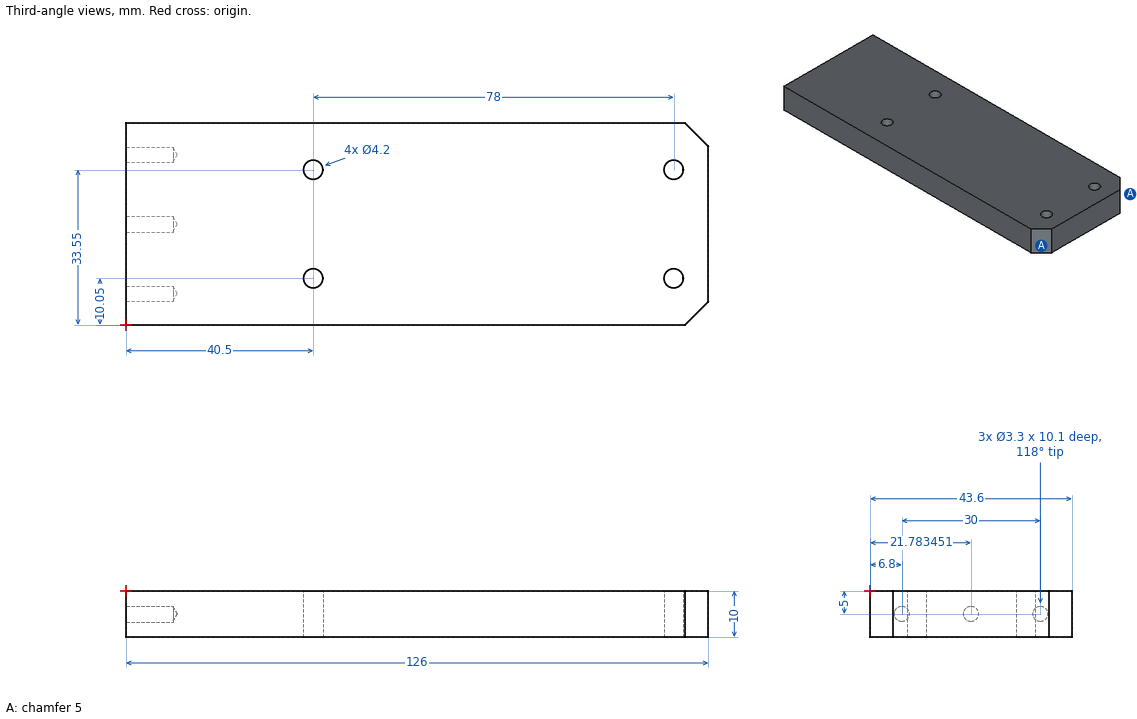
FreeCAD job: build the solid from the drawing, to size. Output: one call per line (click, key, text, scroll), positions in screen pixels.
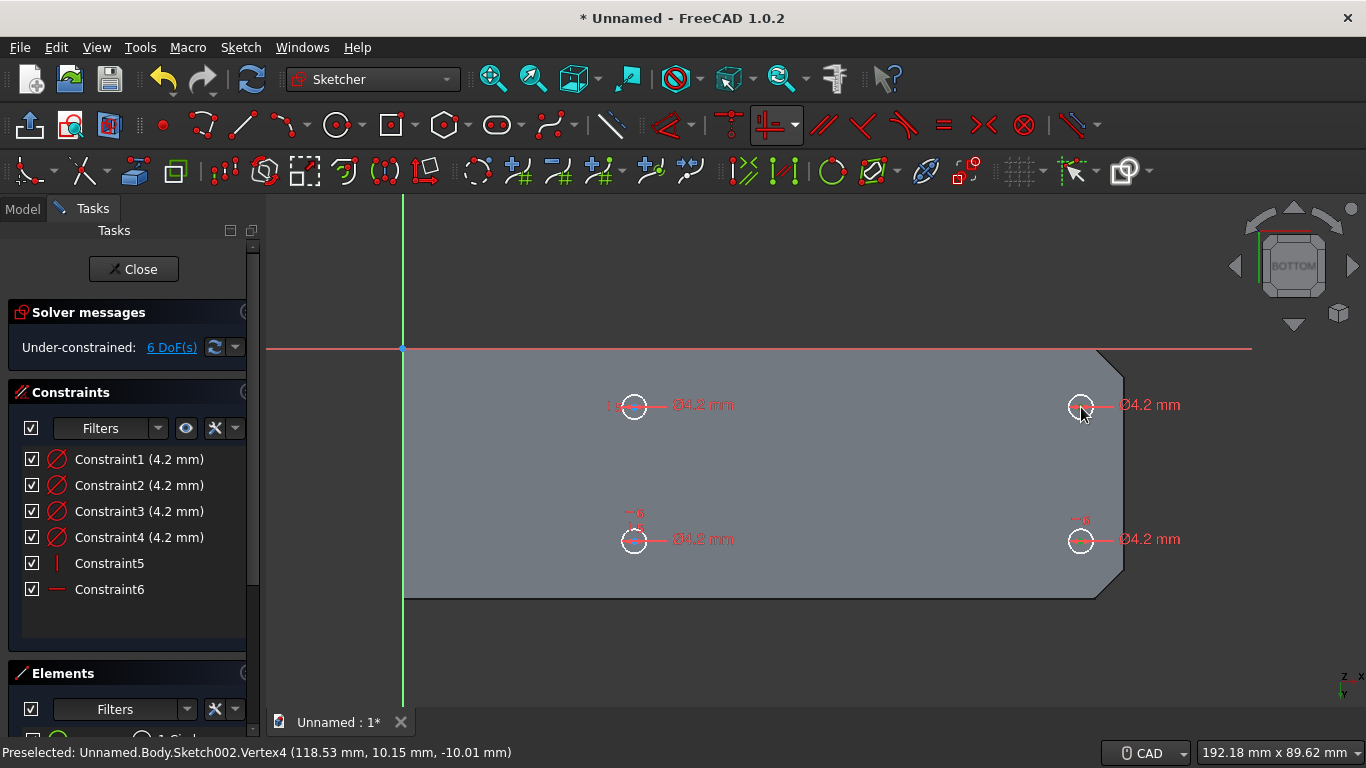
key(v)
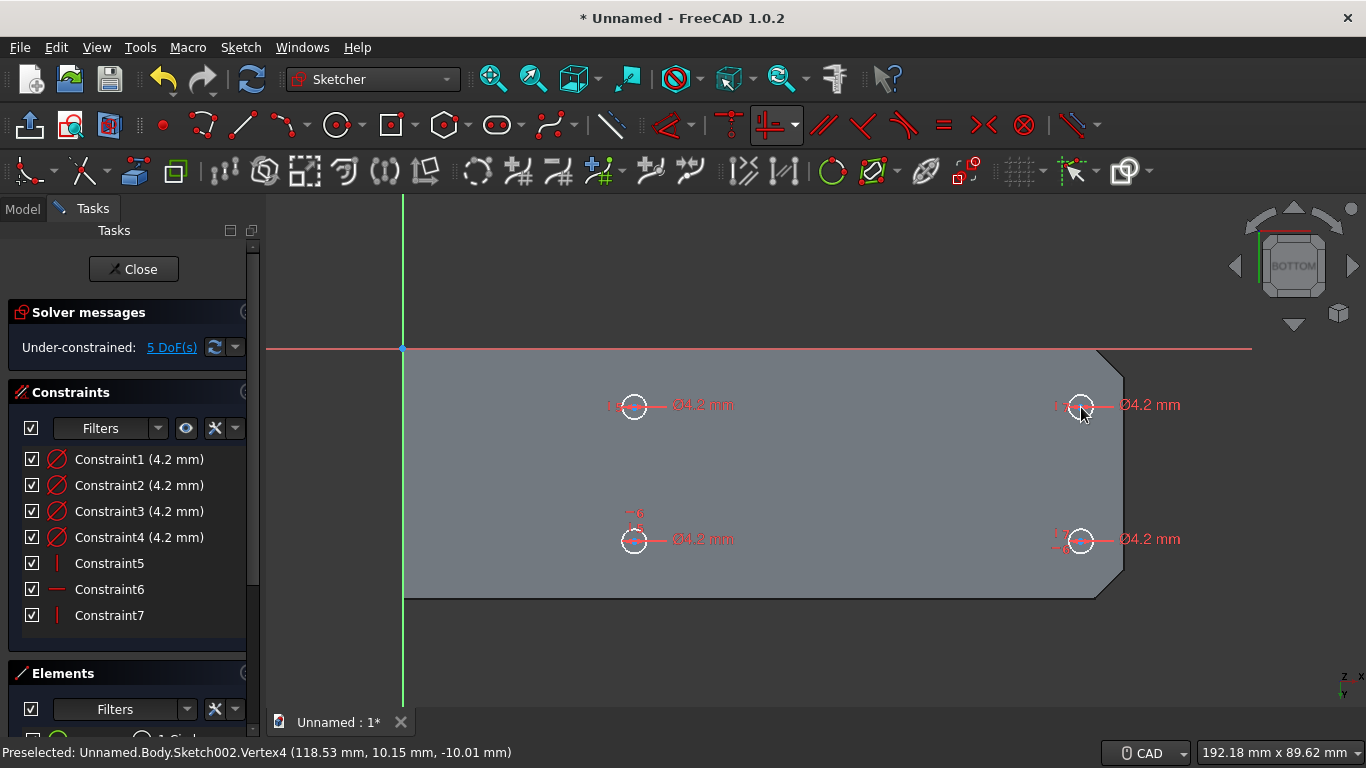
click(634, 407)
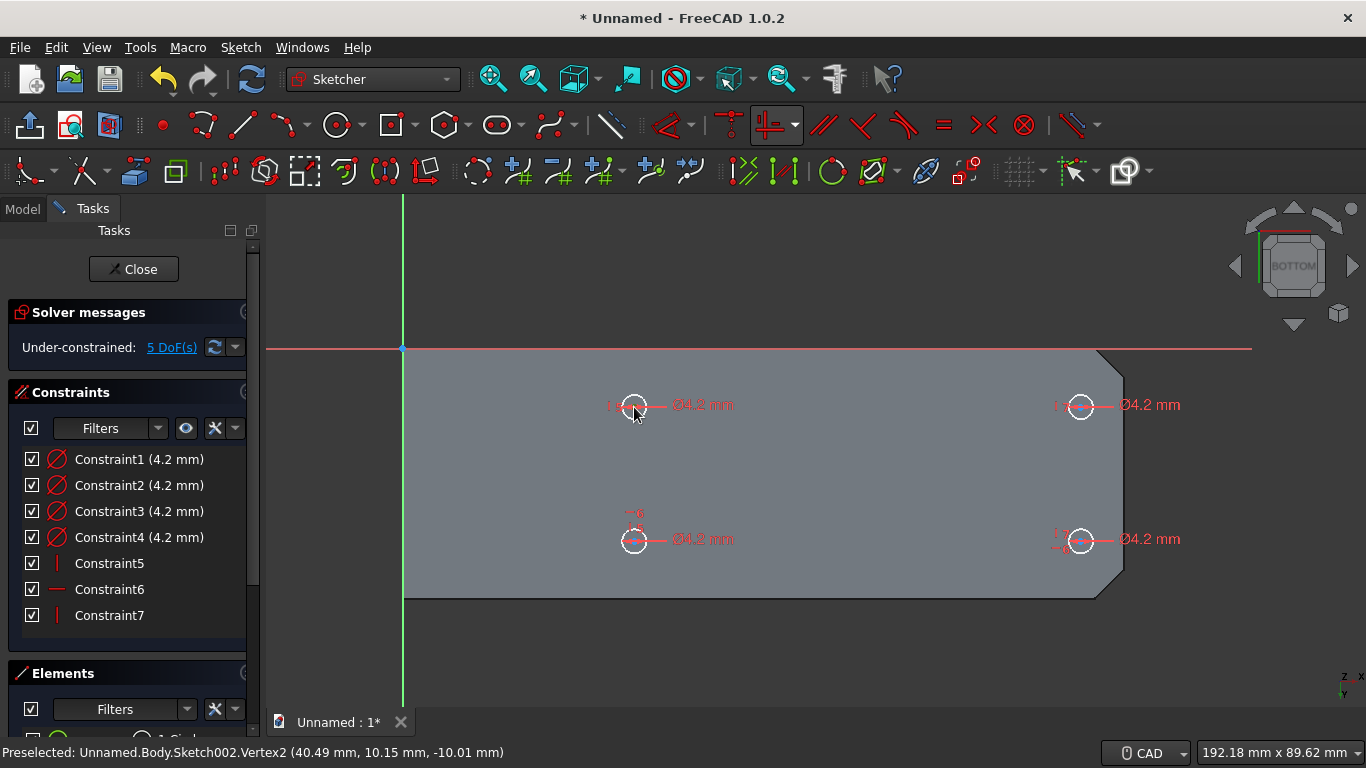
click(1081, 407)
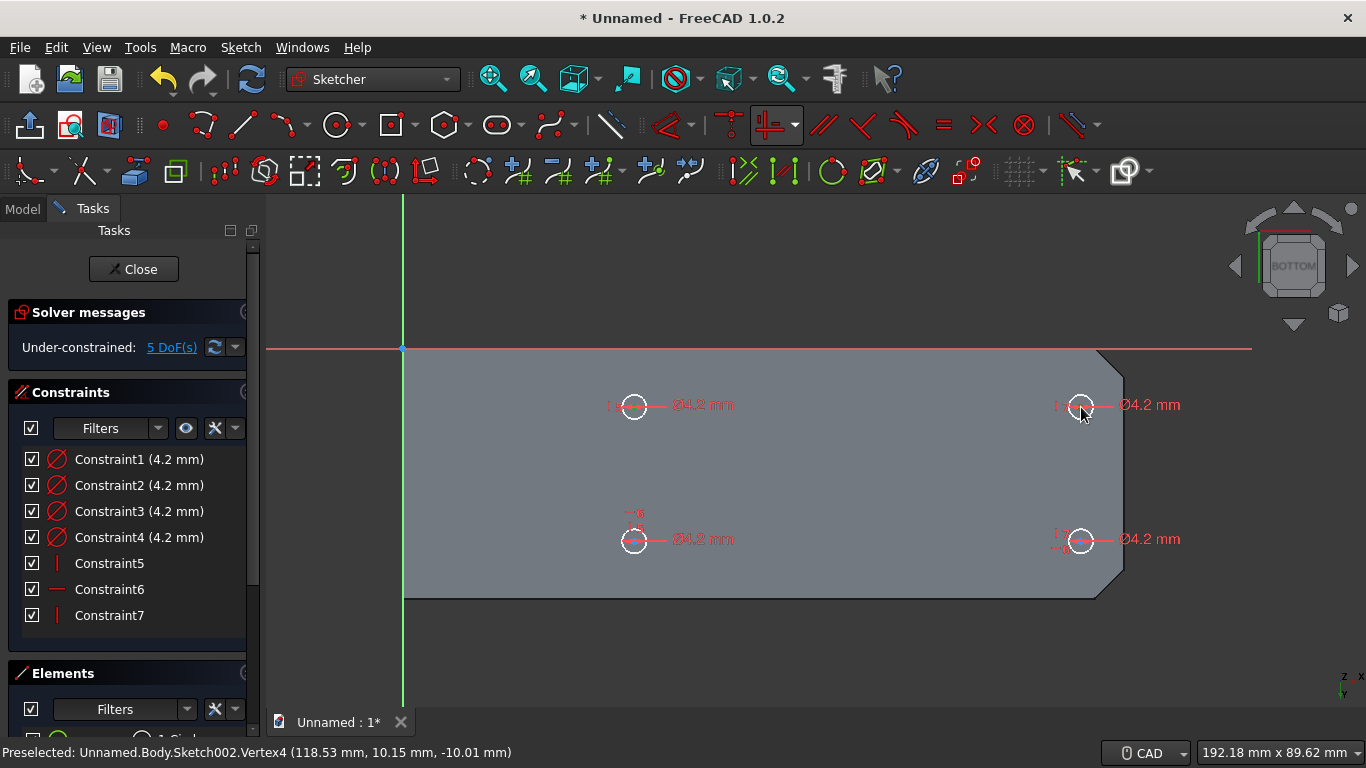
click(798, 126)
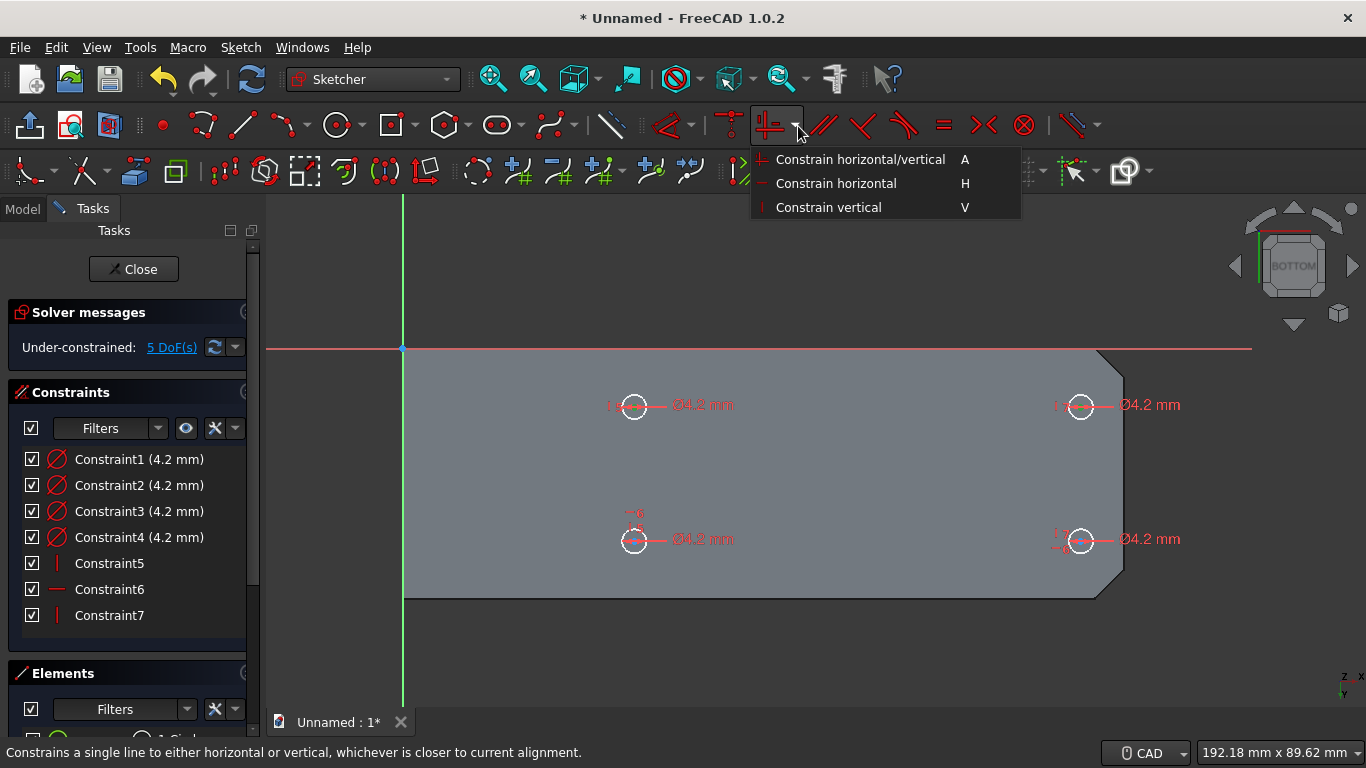
click(886, 183)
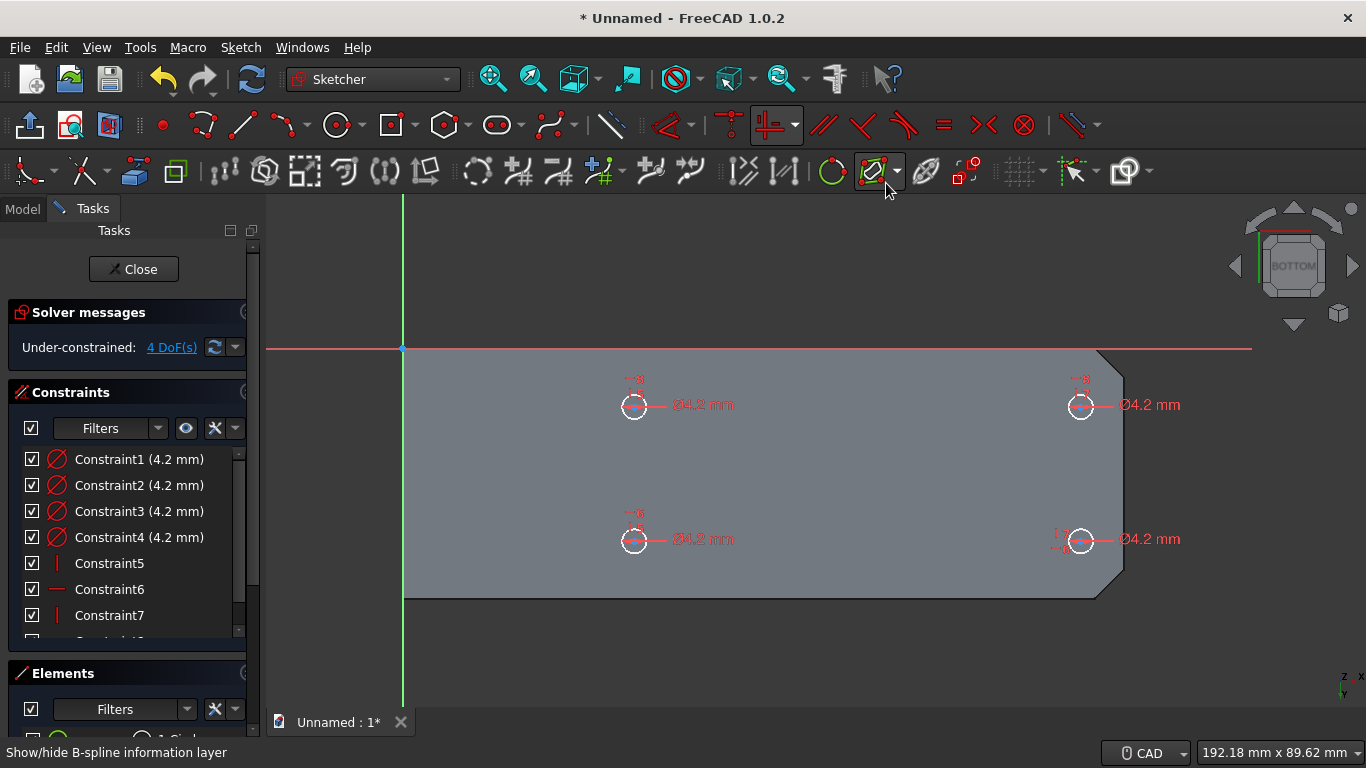
click(666, 126)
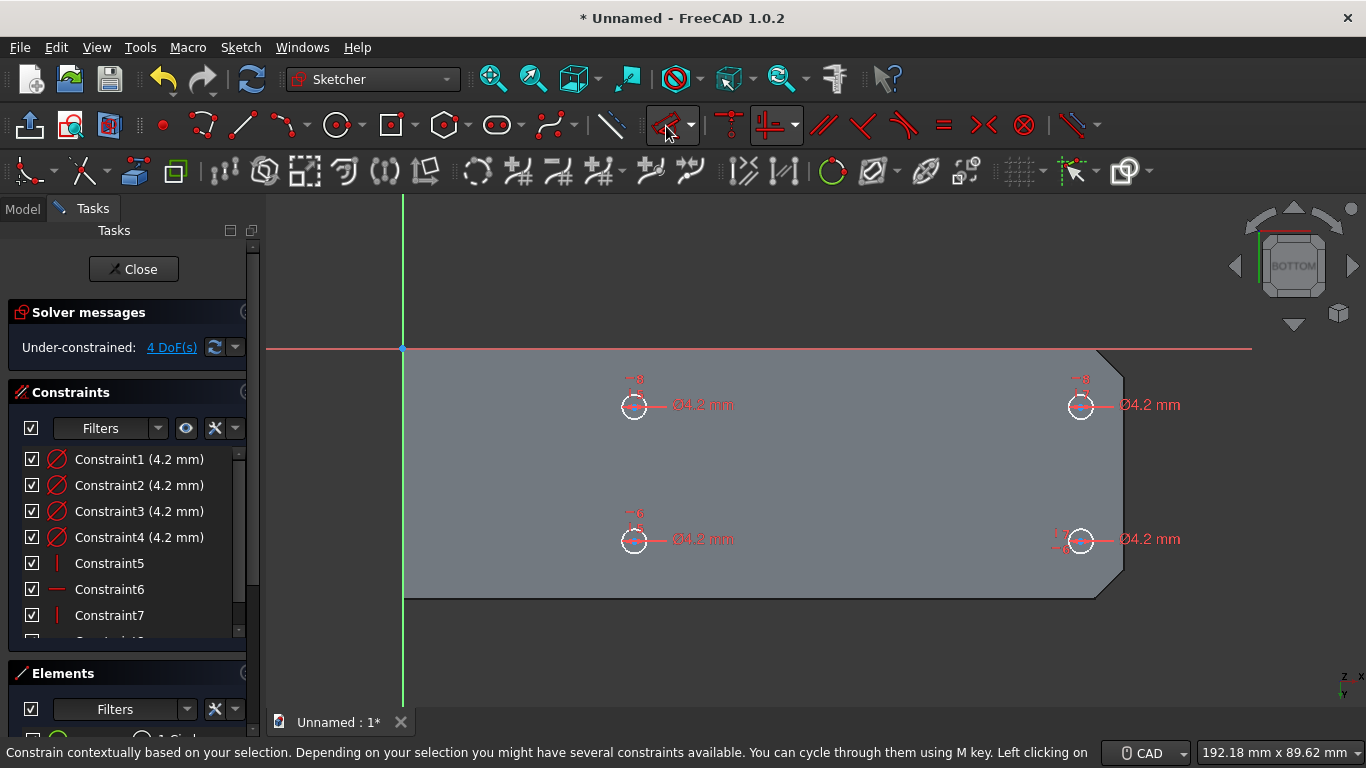
click(634, 541)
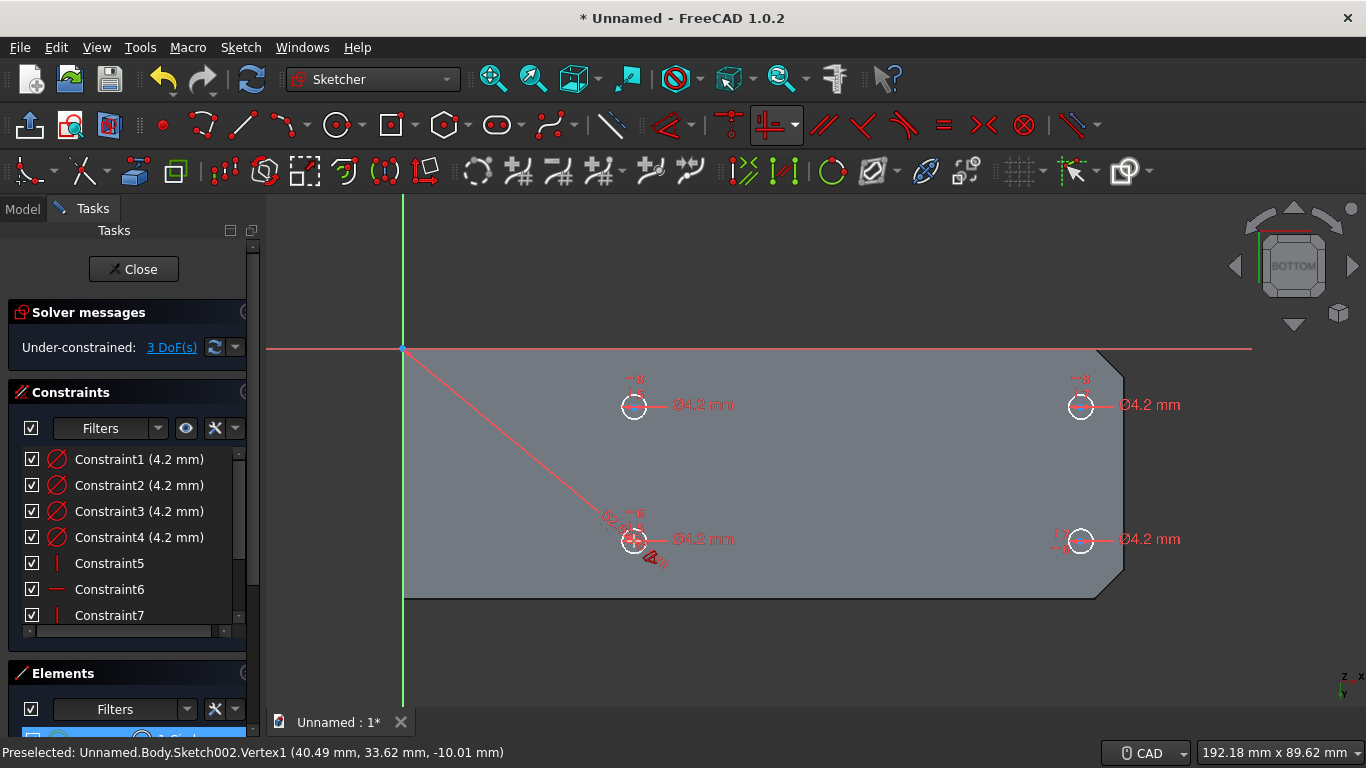
click(1081, 541)
click(858, 575)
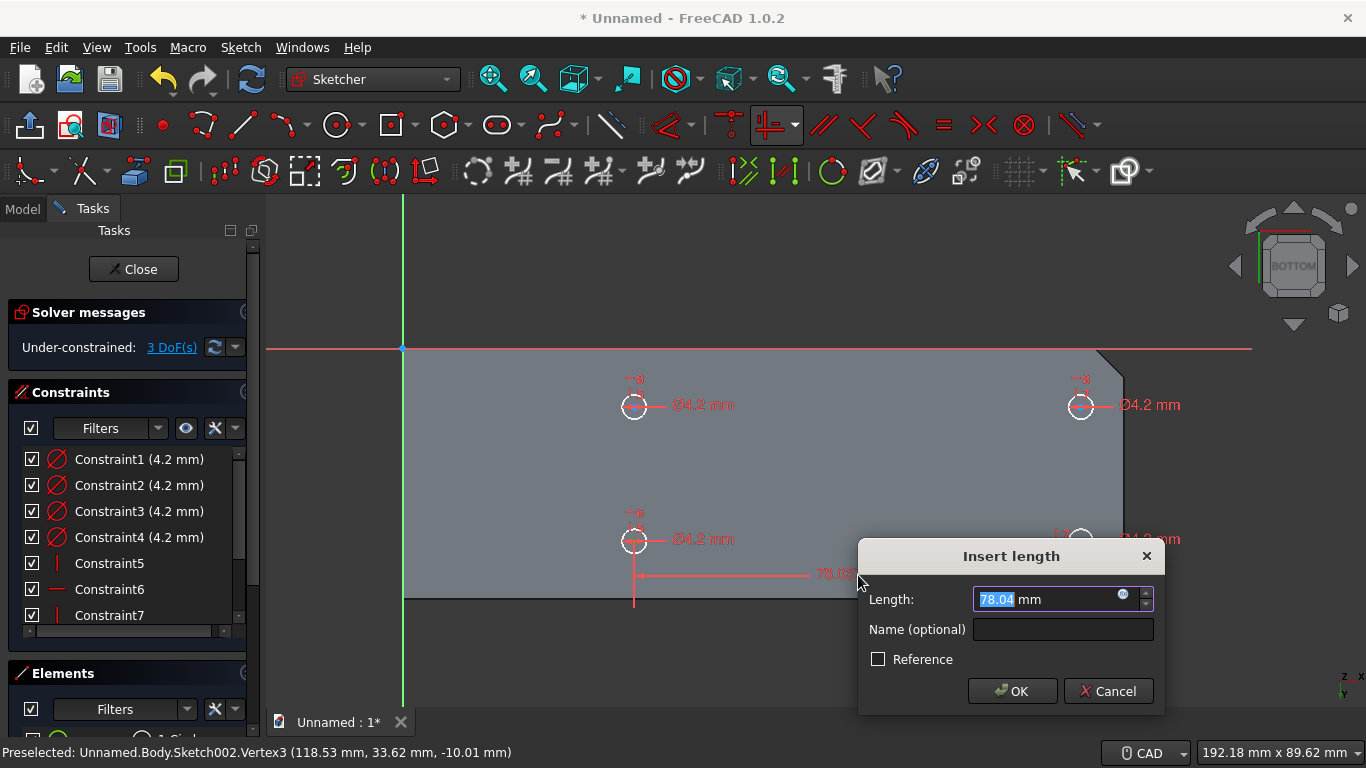
text(78)
key(Return)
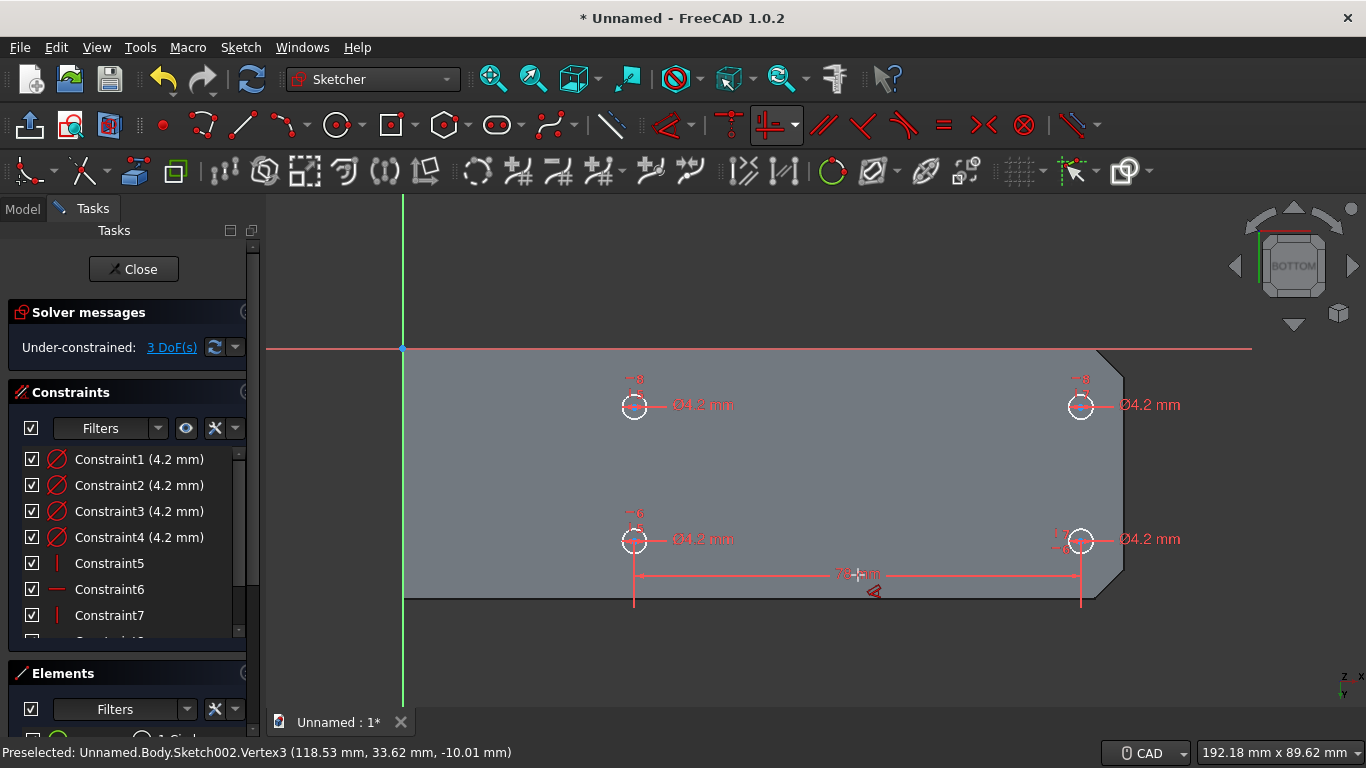
click(634, 541)
click(519, 315)